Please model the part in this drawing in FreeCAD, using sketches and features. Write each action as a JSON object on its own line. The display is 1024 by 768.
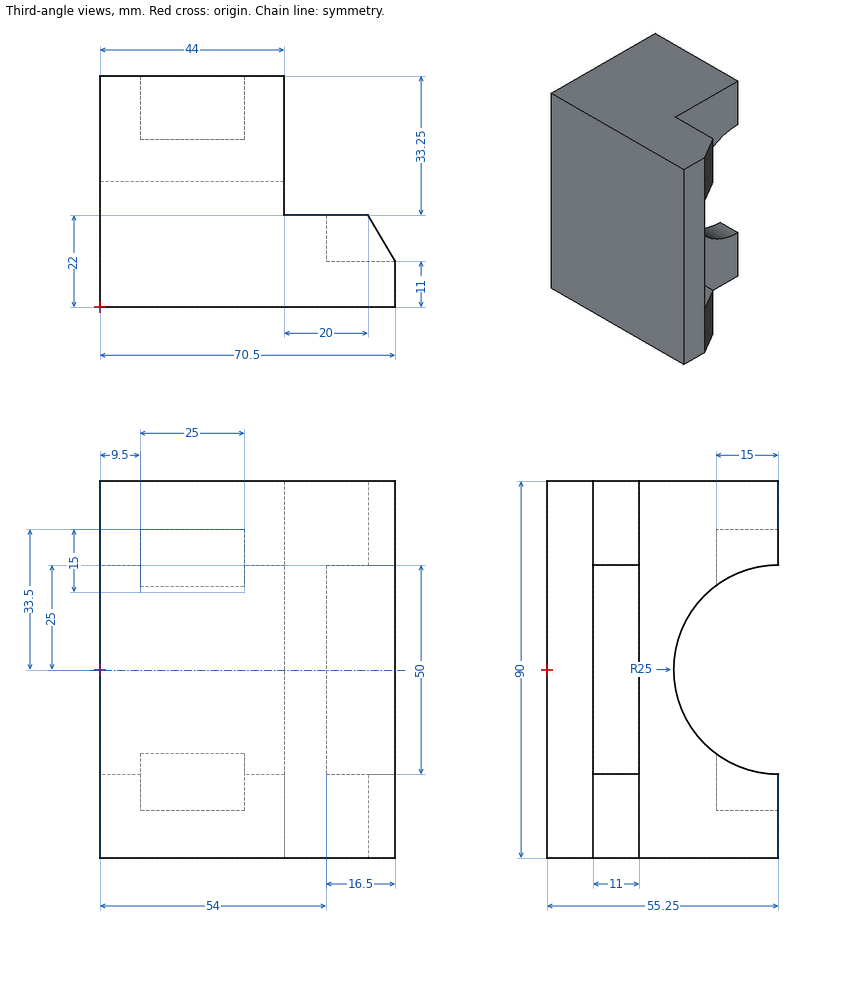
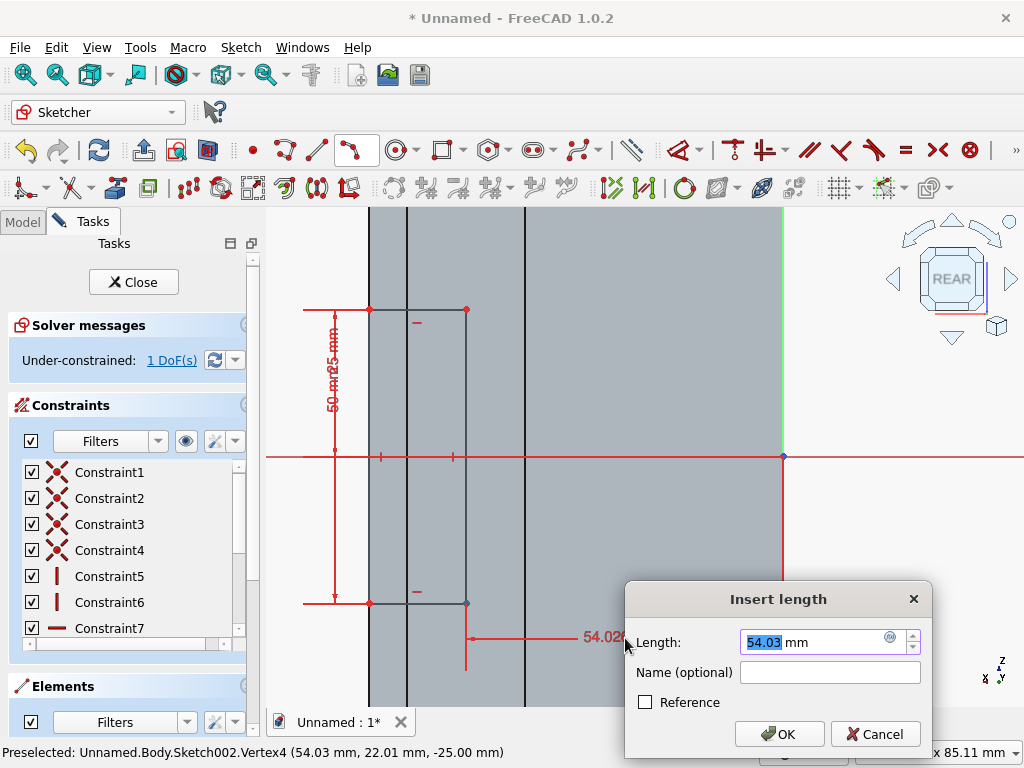
{"action": "type", "text": "54"}
{"action": "key", "text": "Return"}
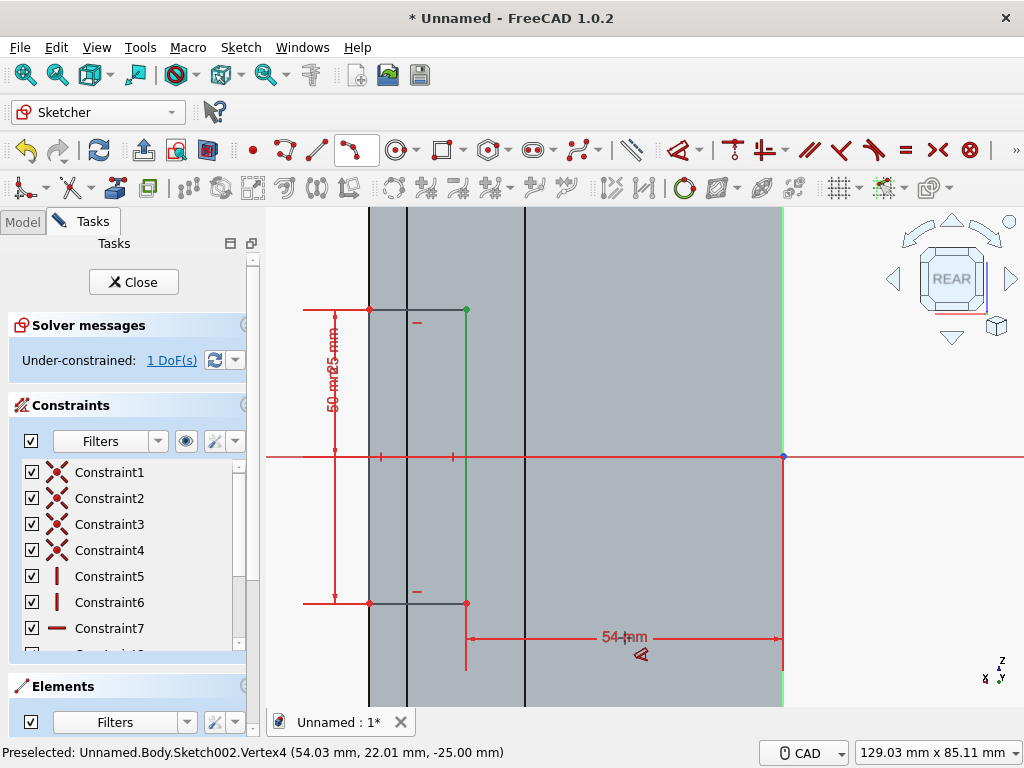
{"action": "left_click", "coordinate": [398, 604]}
{"action": "left_click", "coordinate": [418, 638]}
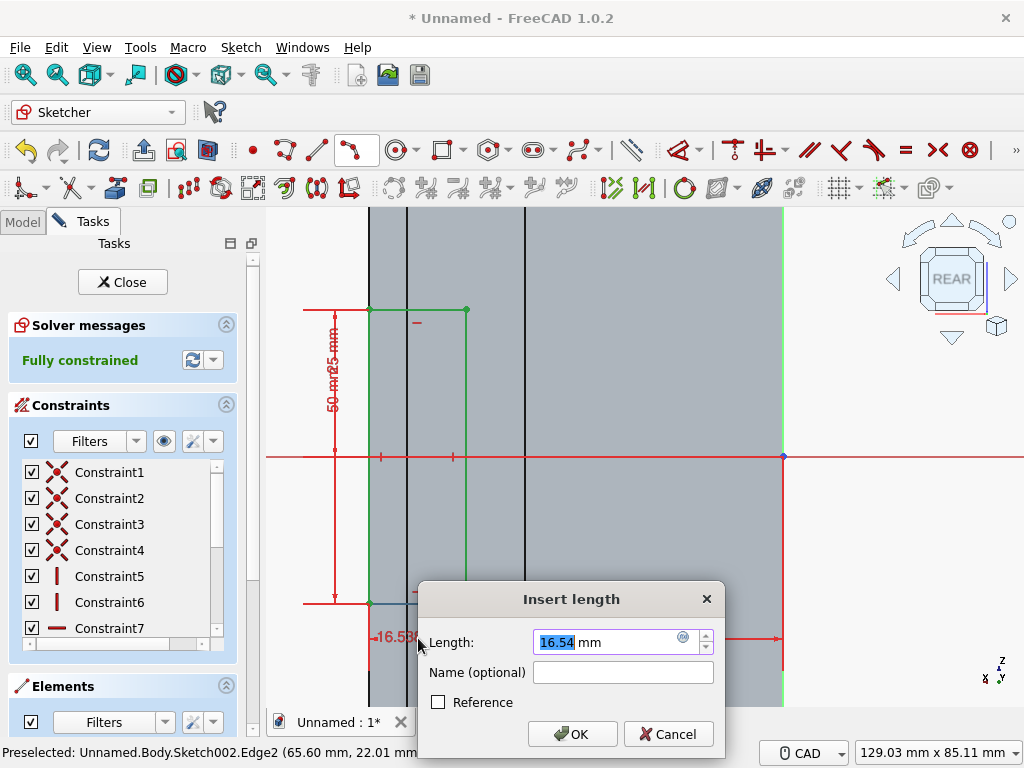
{"action": "type", "text": "16.5"}
{"action": "key", "text": "Return"}
{"action": "key", "text": "Escape"}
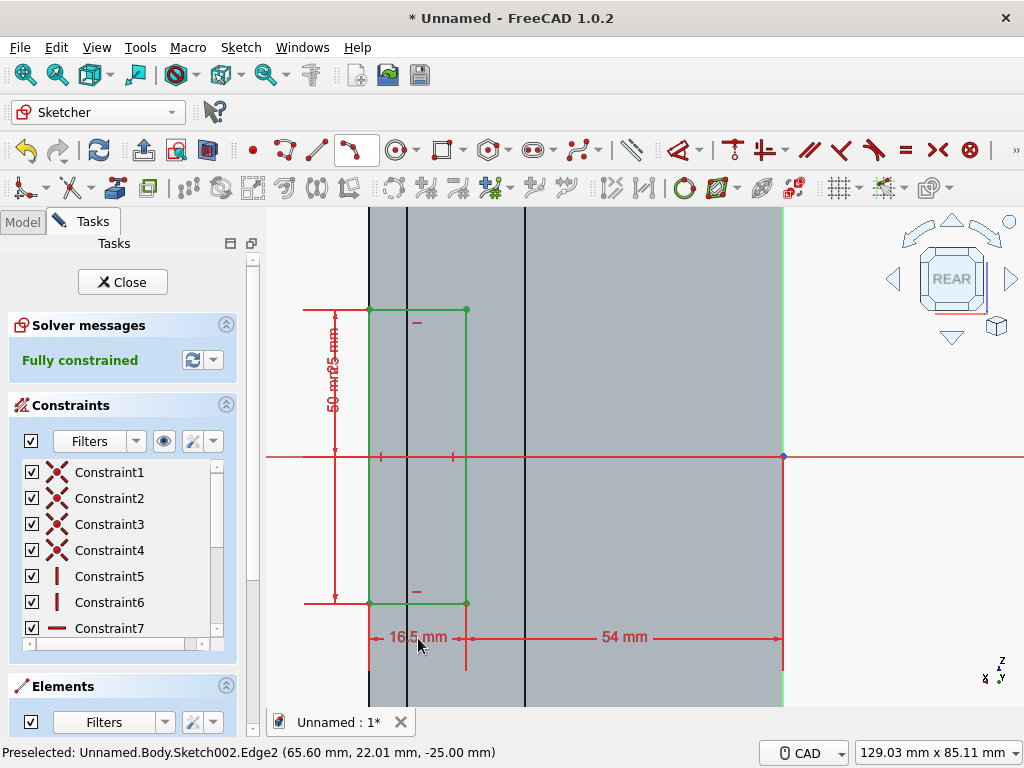
{"action": "left_click", "coordinate": [123, 282]}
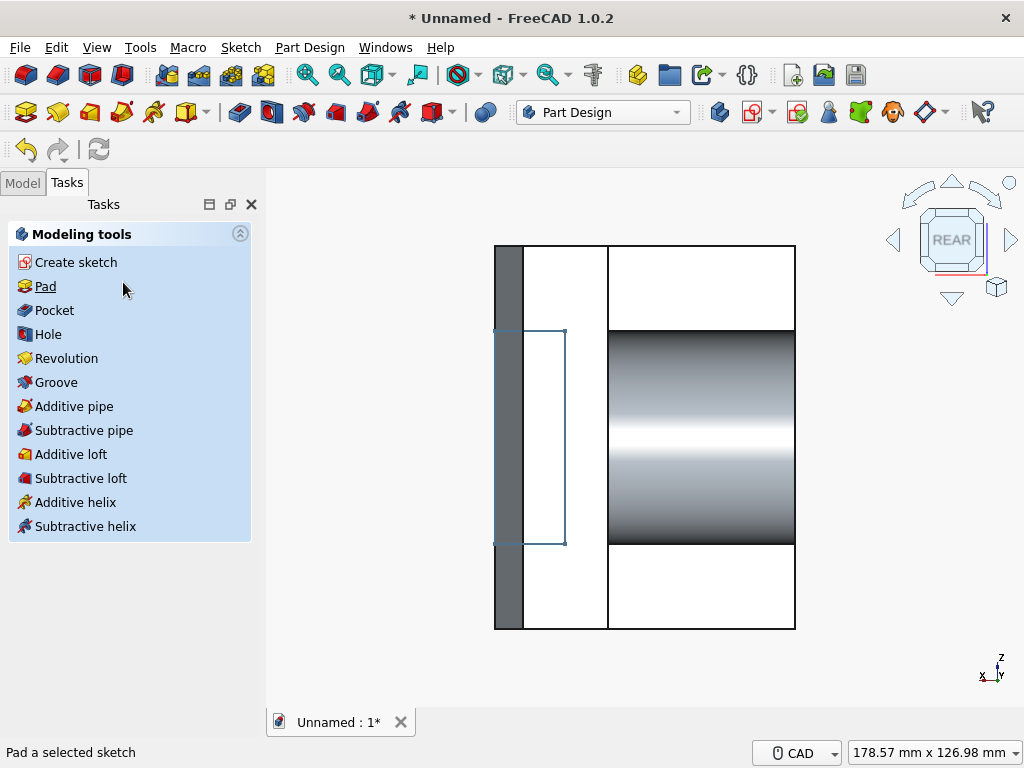
{"action": "left_click", "coordinate": [240, 112]}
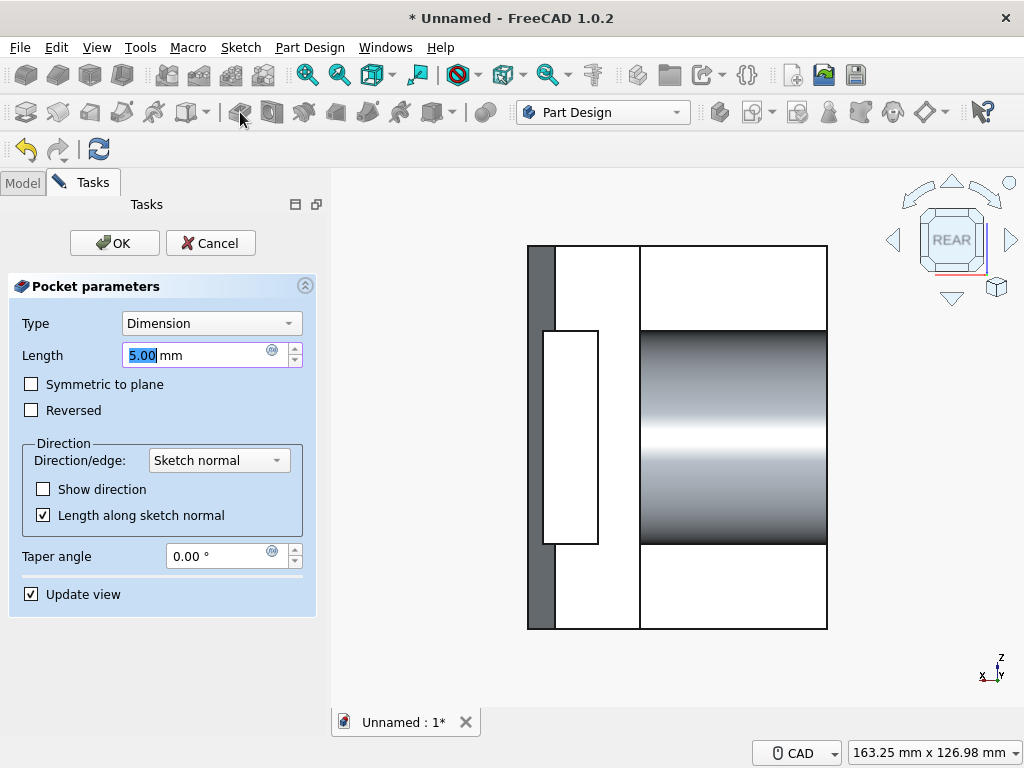
{"action": "type", "text": "11"}
{"action": "key", "text": "Tab"}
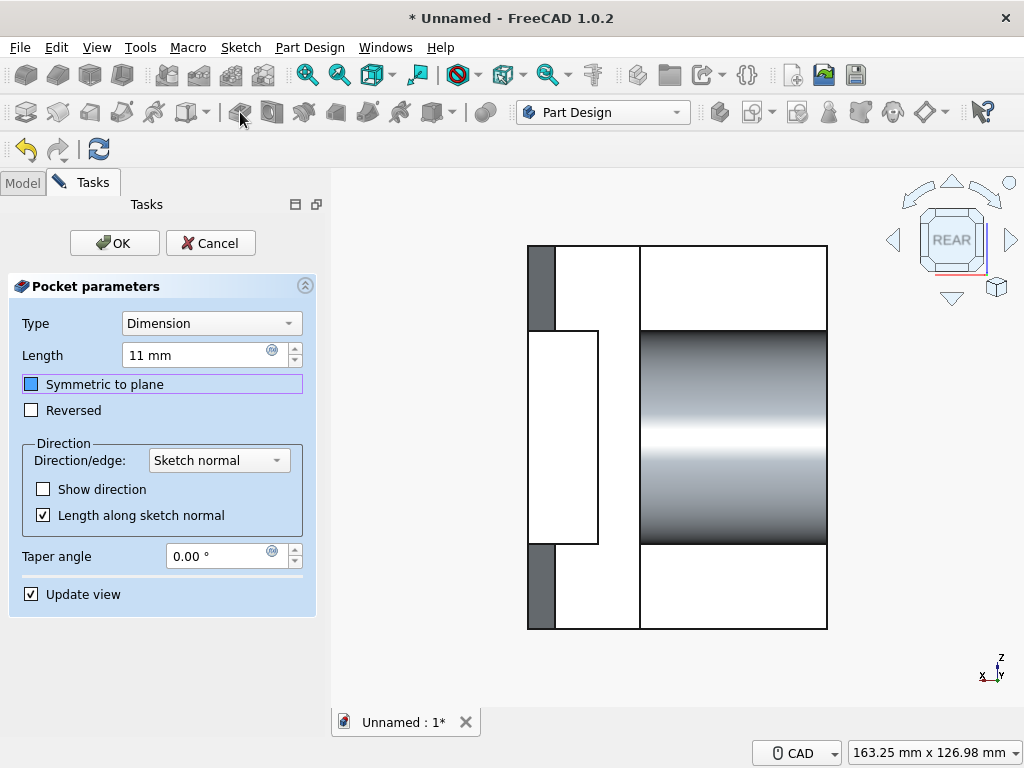
{"action": "left_click", "coordinate": [115, 243]}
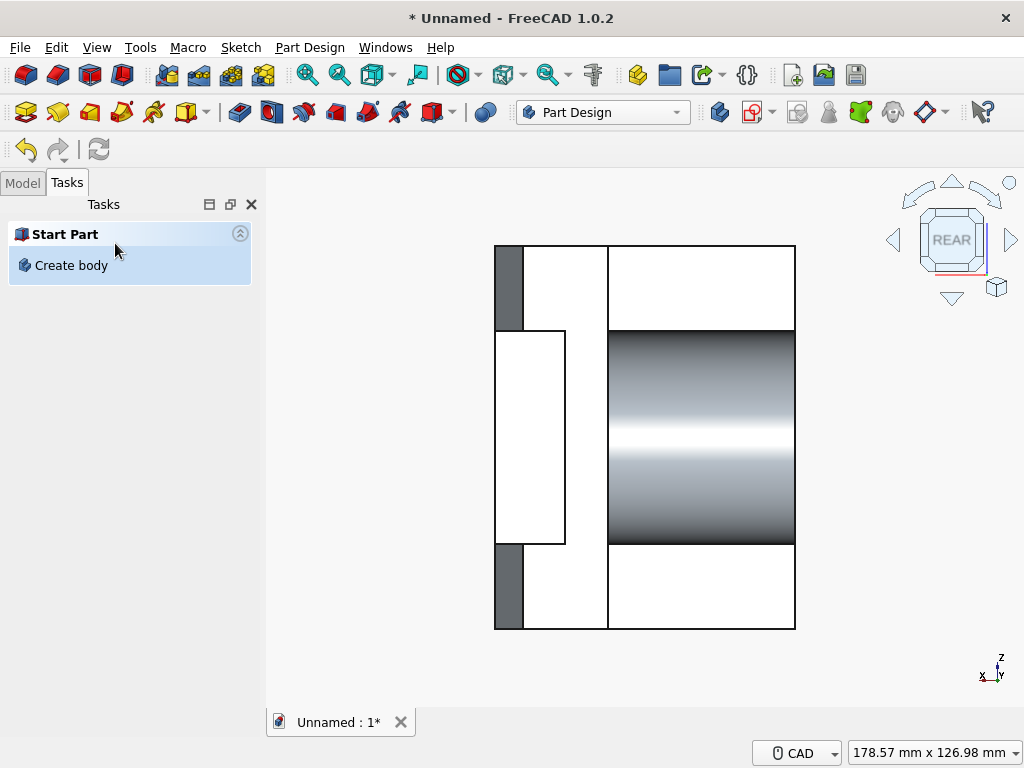
{"action": "left_click", "coordinate": [675, 585]}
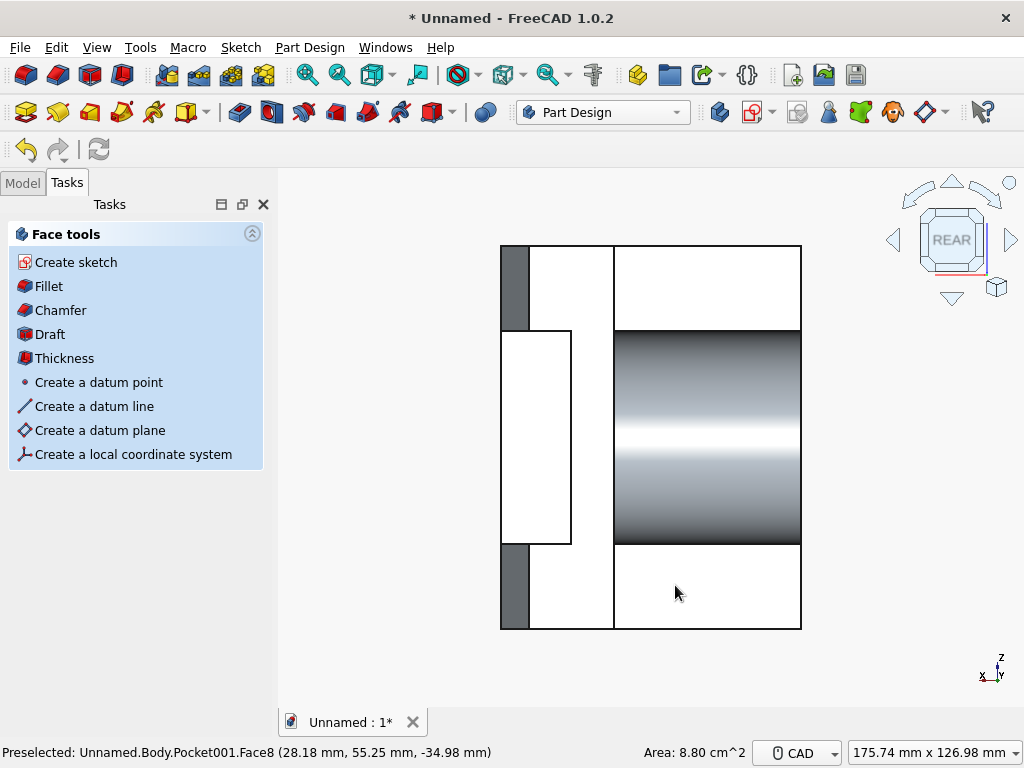
{"action": "left_click", "coordinate": [752, 112]}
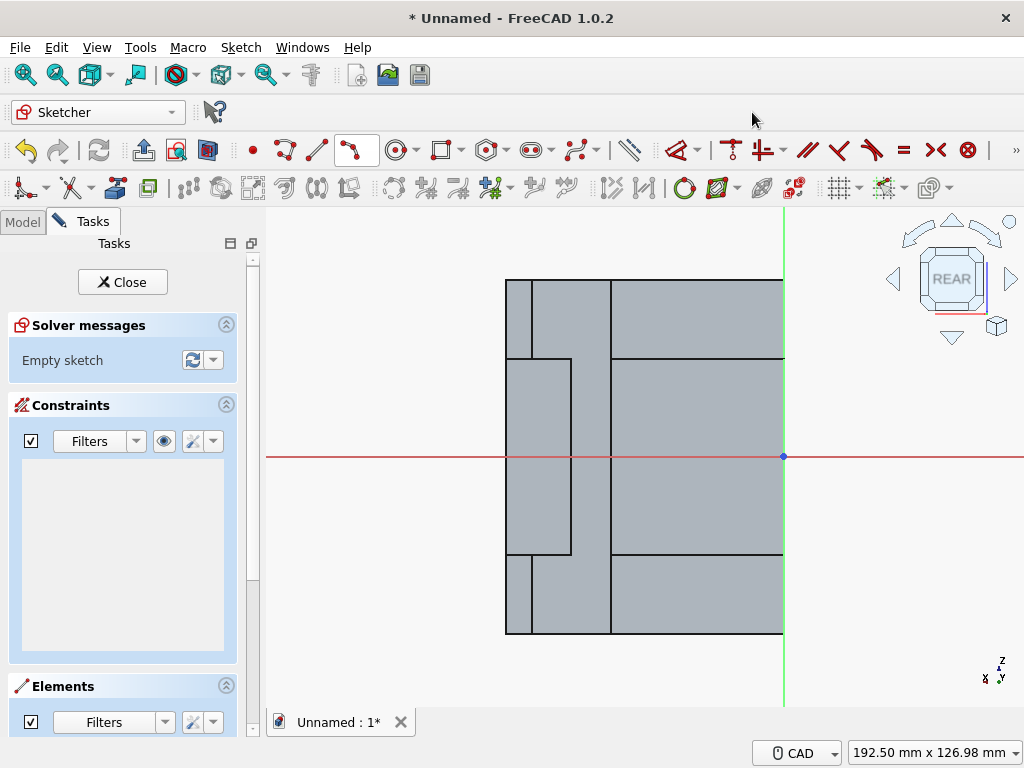
{"action": "left_click", "coordinate": [442, 150]}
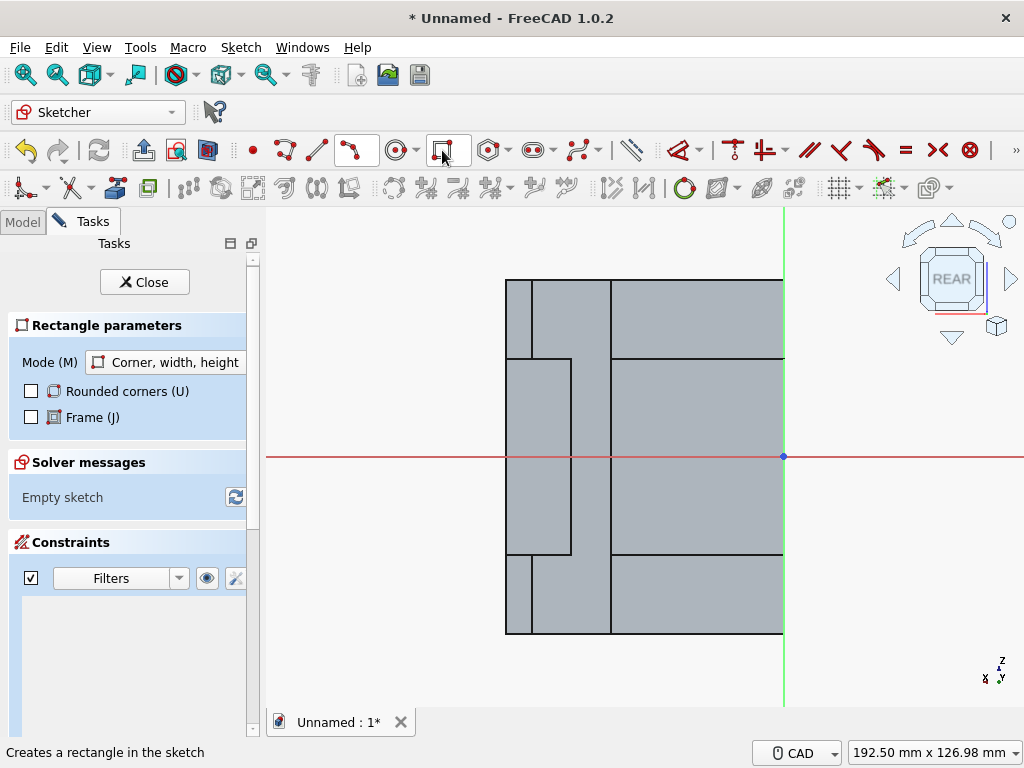
{"action": "left_click", "coordinate": [648, 325]}
{"action": "left_click", "coordinate": [746, 384]}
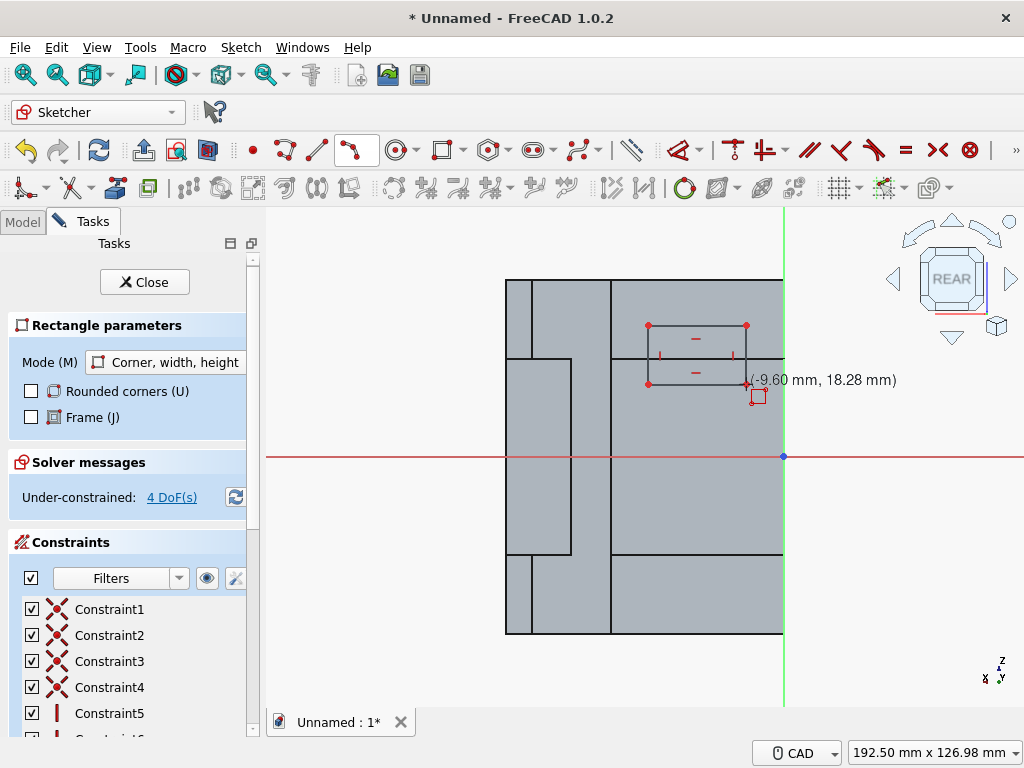
{"action": "left_click", "coordinate": [648, 530]}
{"action": "left_click", "coordinate": [746, 589]}
{"action": "key", "text": "Escape"}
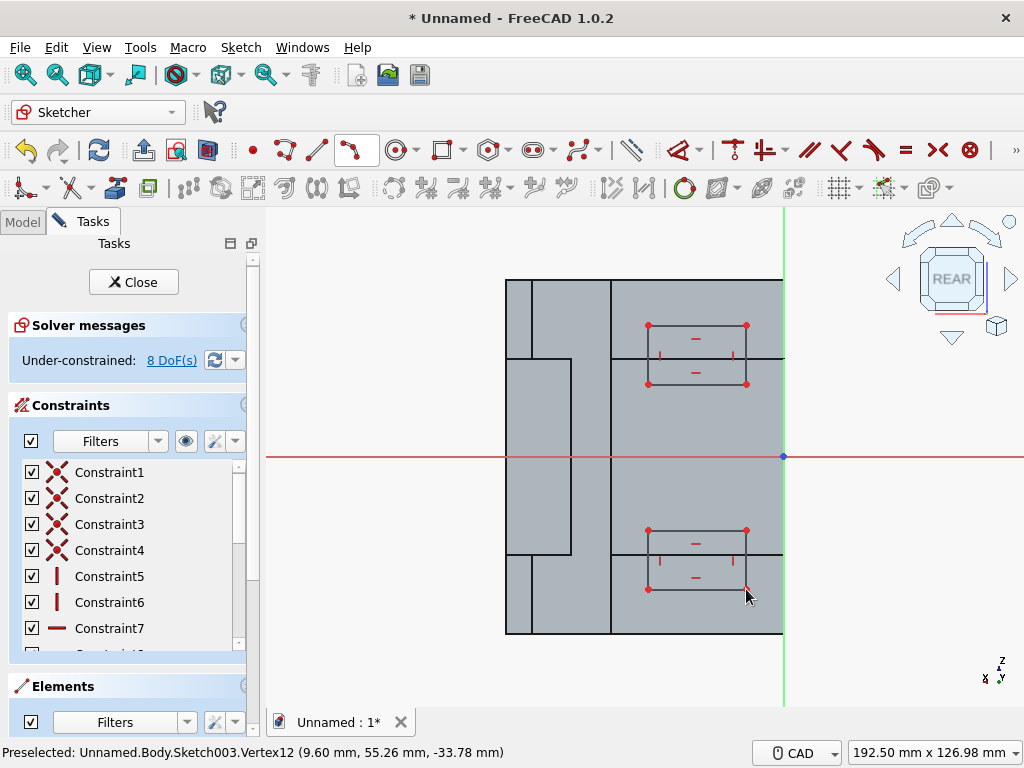
{"action": "left_click", "coordinate": [648, 385]}